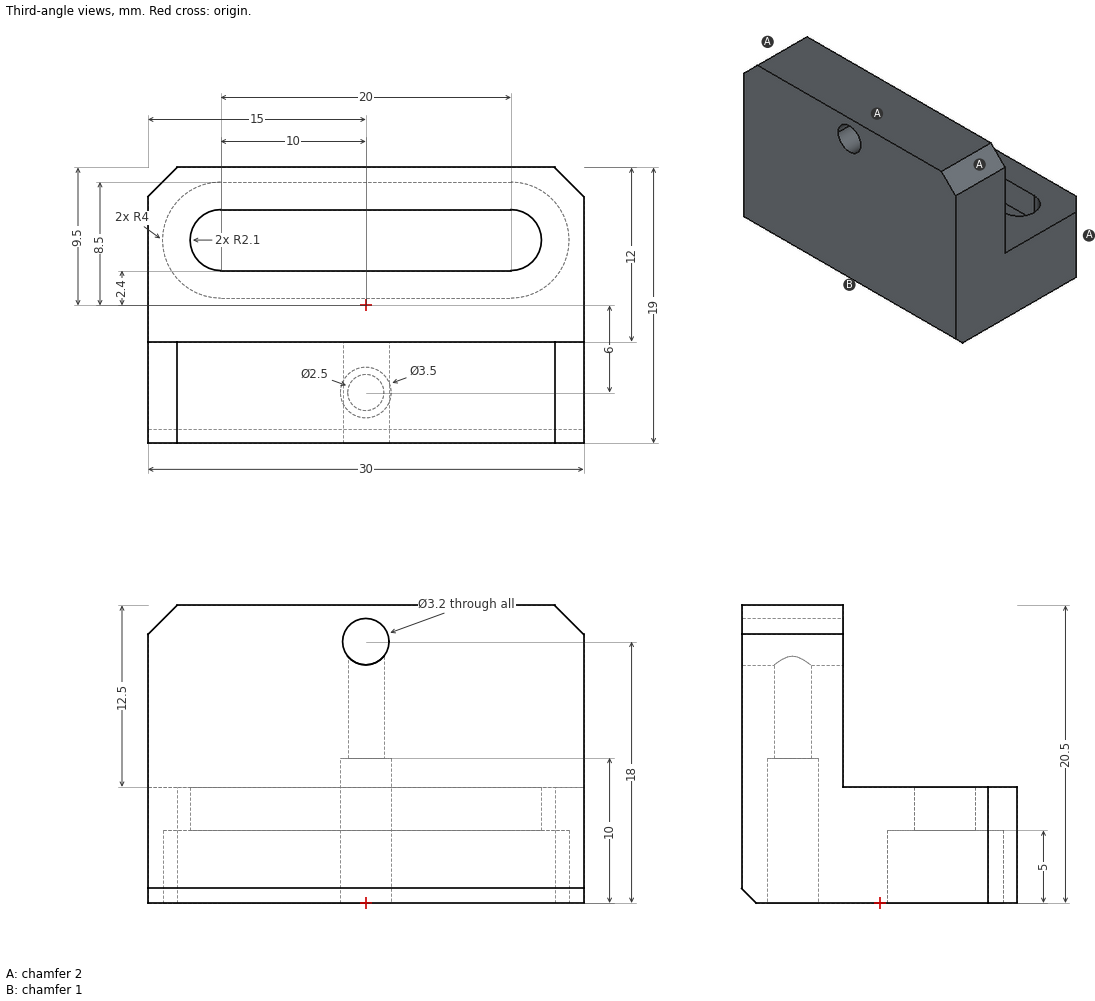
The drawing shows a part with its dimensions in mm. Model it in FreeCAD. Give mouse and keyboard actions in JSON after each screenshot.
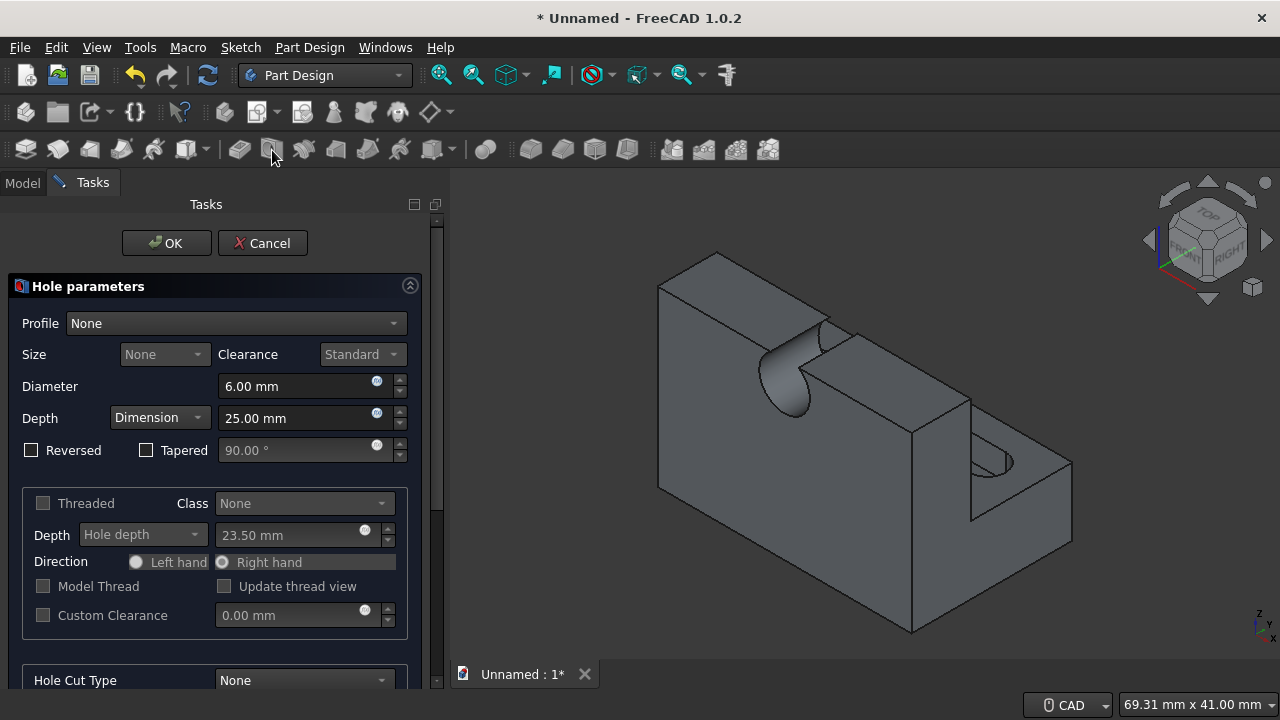
{"action": "triple_click", "coordinate": [305, 386]}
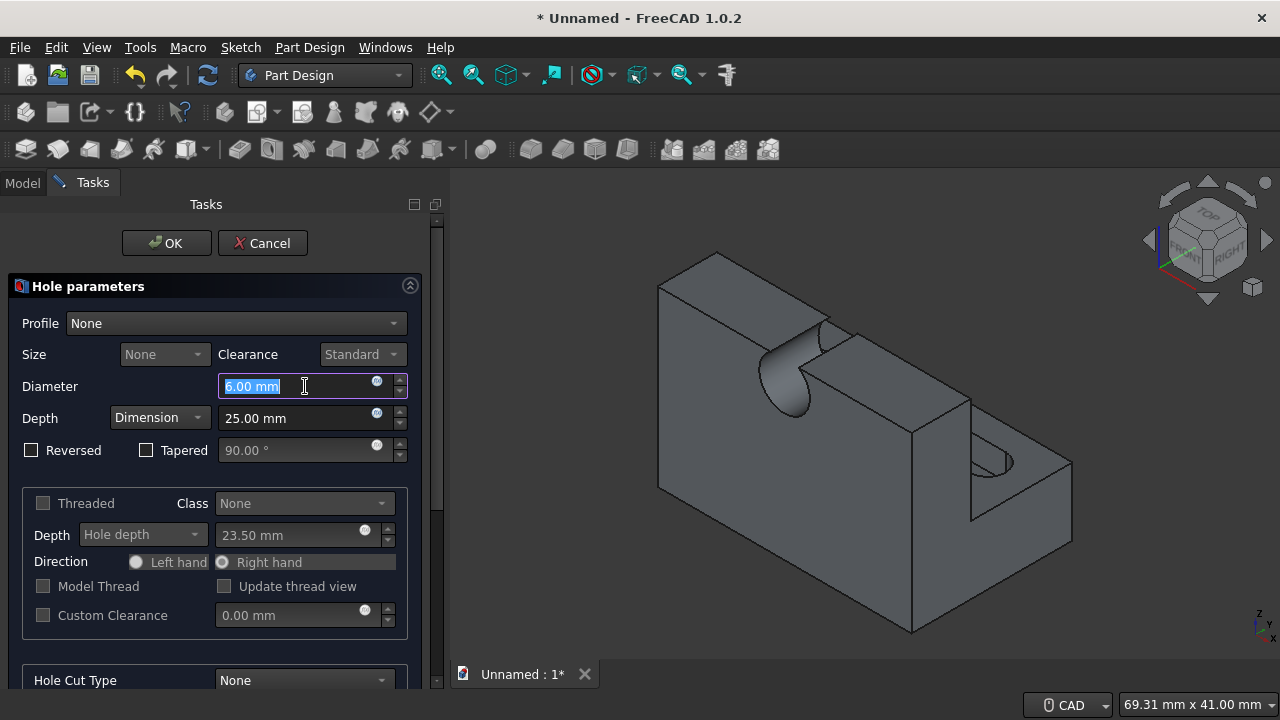
{"action": "type", "text": "3.2"}
{"action": "key", "text": "Tab"}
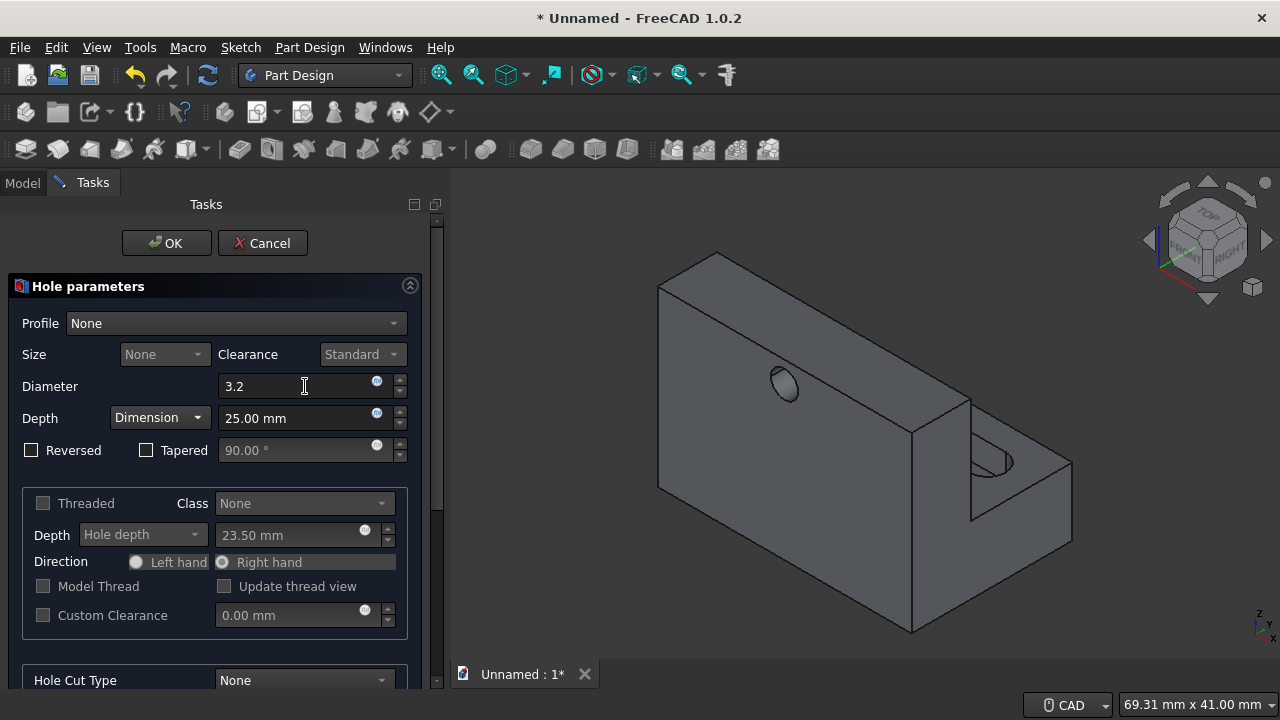
{"action": "left_click", "coordinate": [161, 418]}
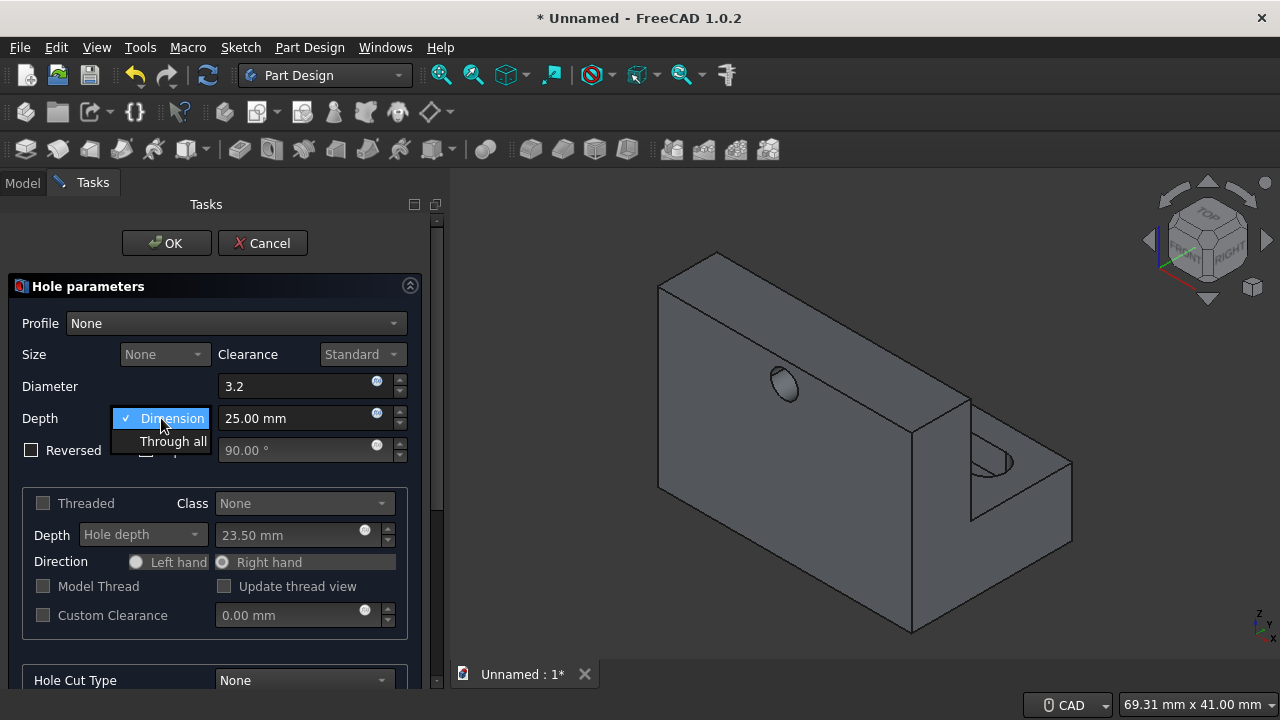
{"action": "left_click", "coordinate": [160, 442]}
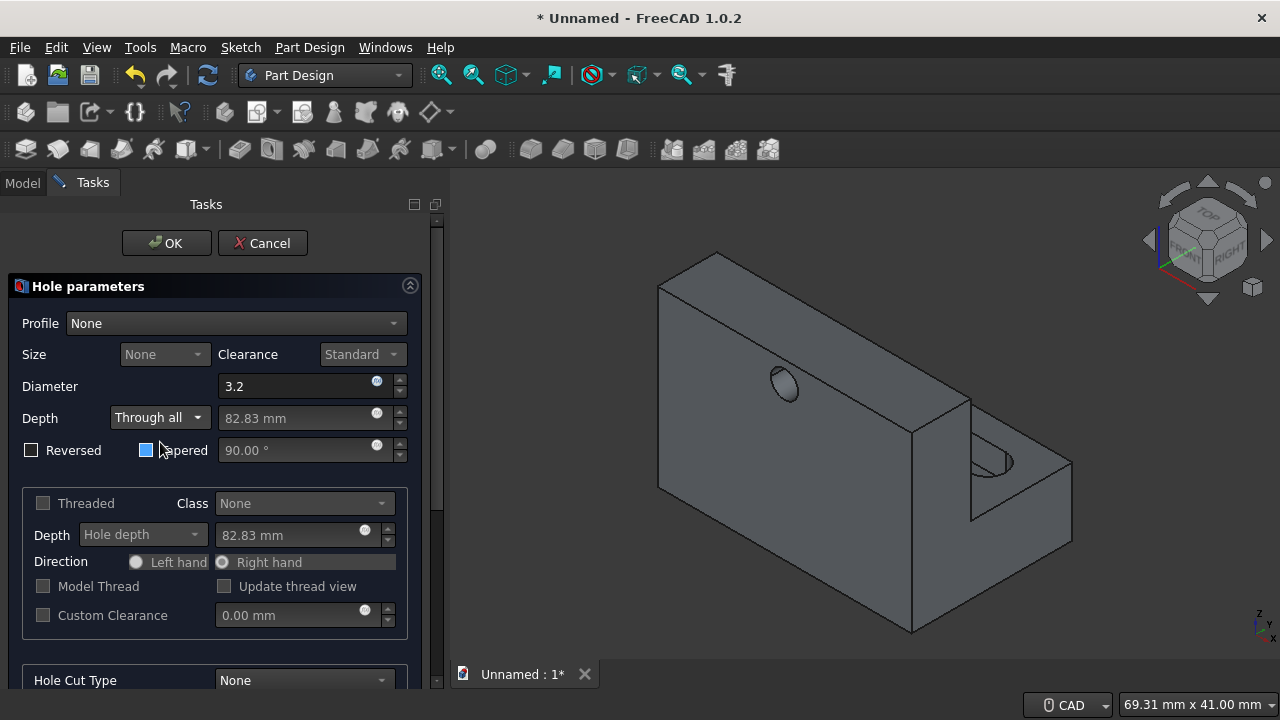
{"action": "left_click", "coordinate": [167, 243]}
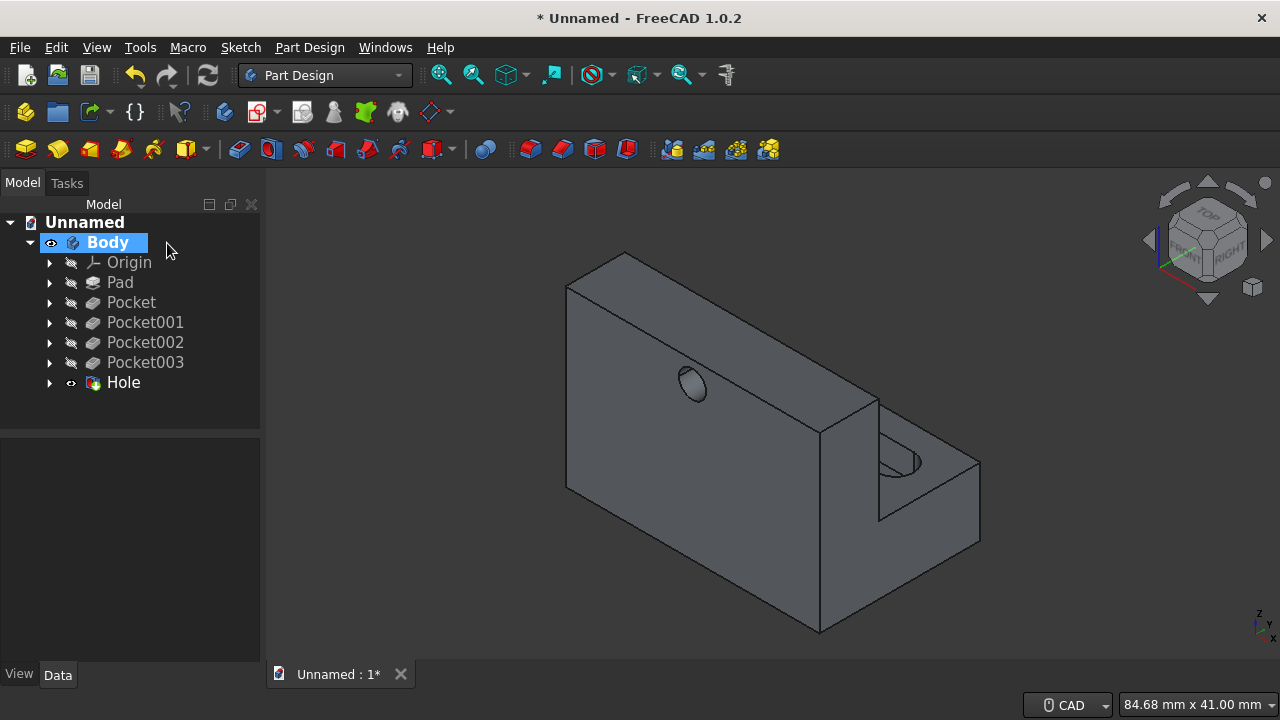
{"action": "key", "text": "5"}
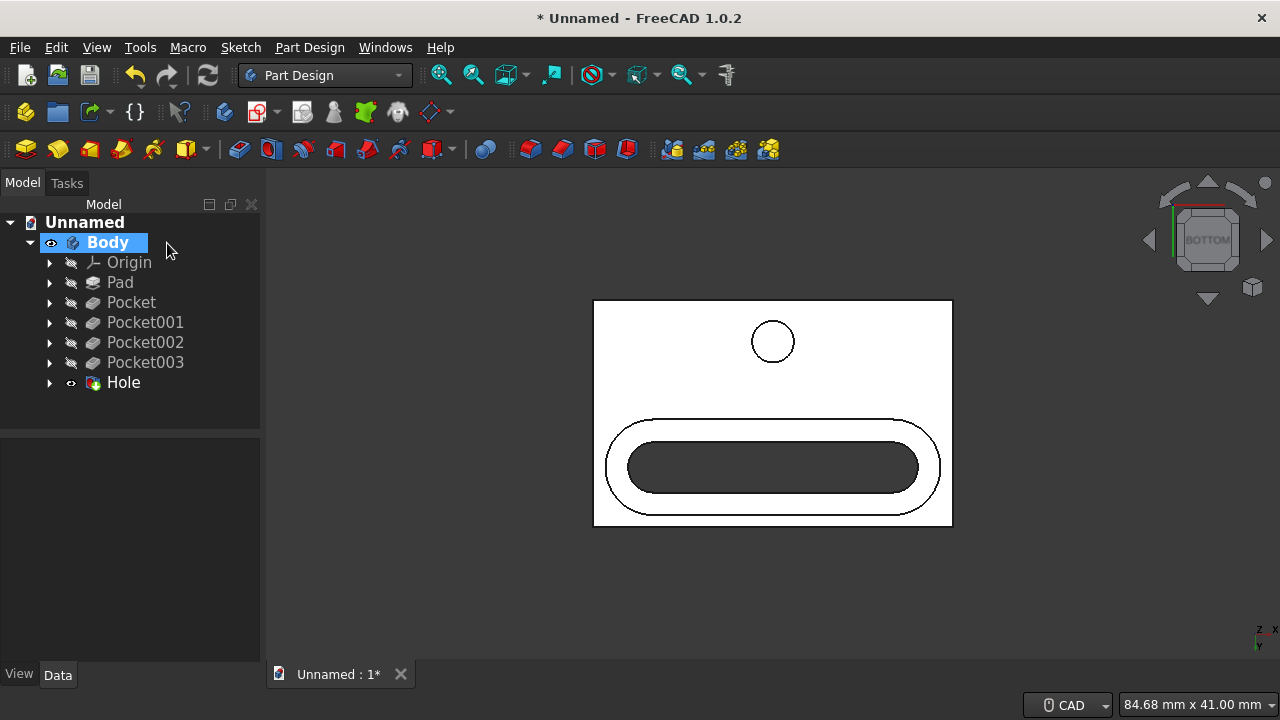
{"action": "left_click", "coordinate": [773, 341]}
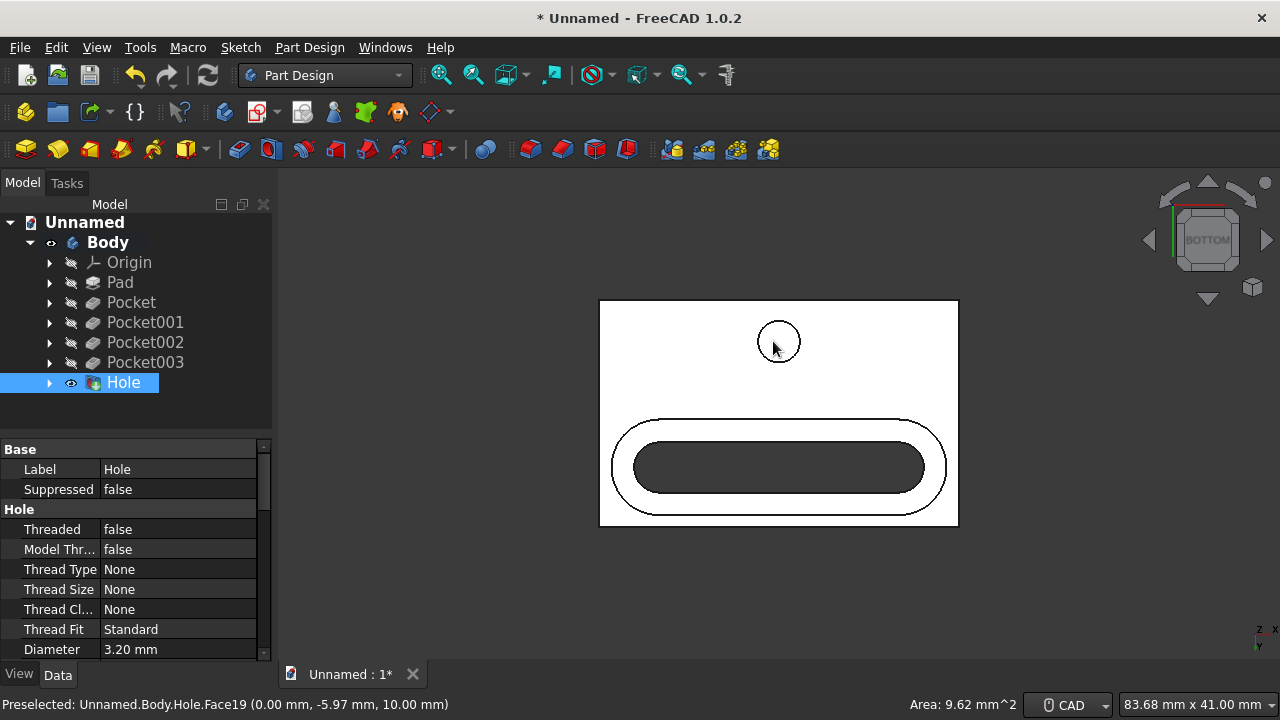
{"action": "left_click", "coordinate": [258, 112]}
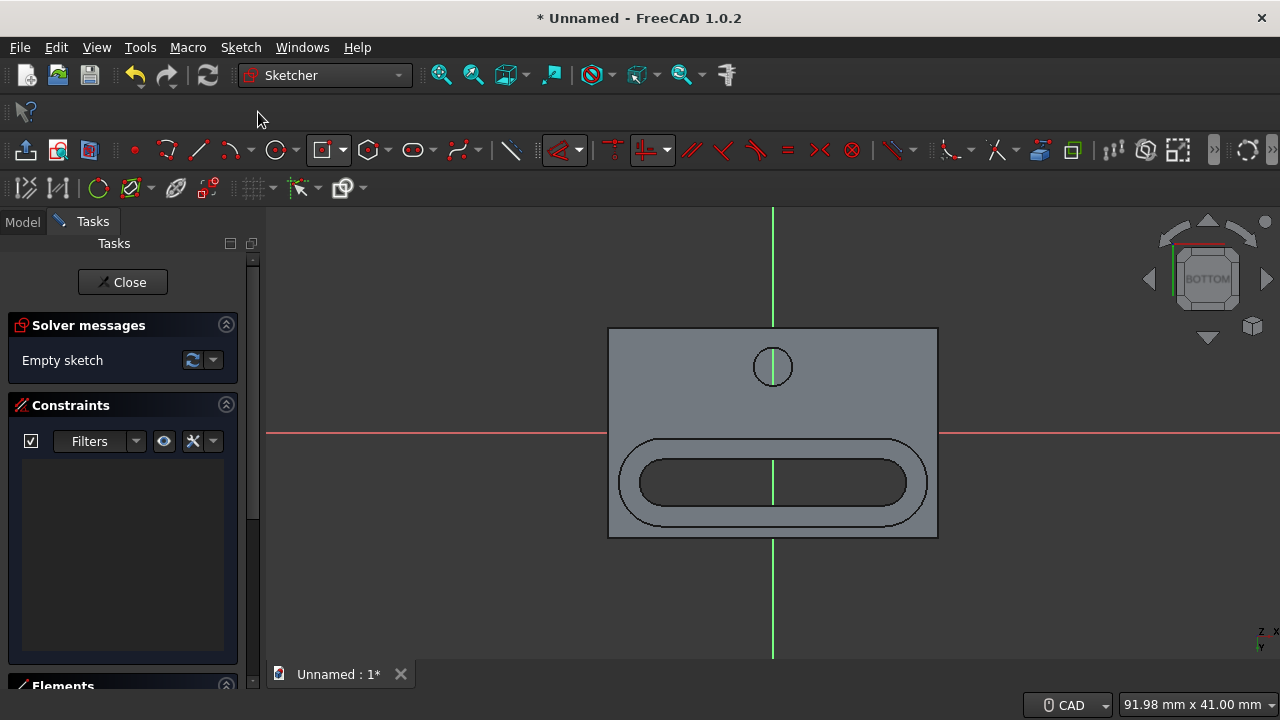
{"action": "left_click", "coordinate": [90, 150]}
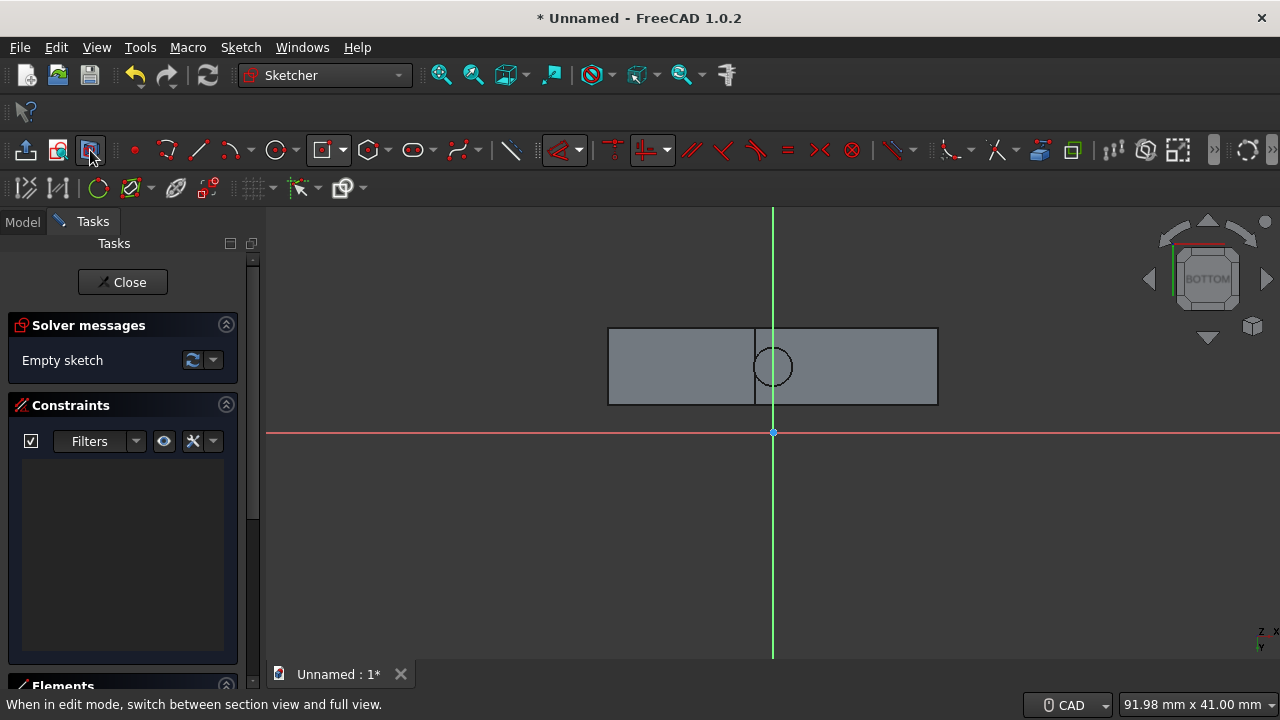
{"action": "scroll", "coordinate": [780, 360], "scroll_direction": "up", "scroll_amount": 12}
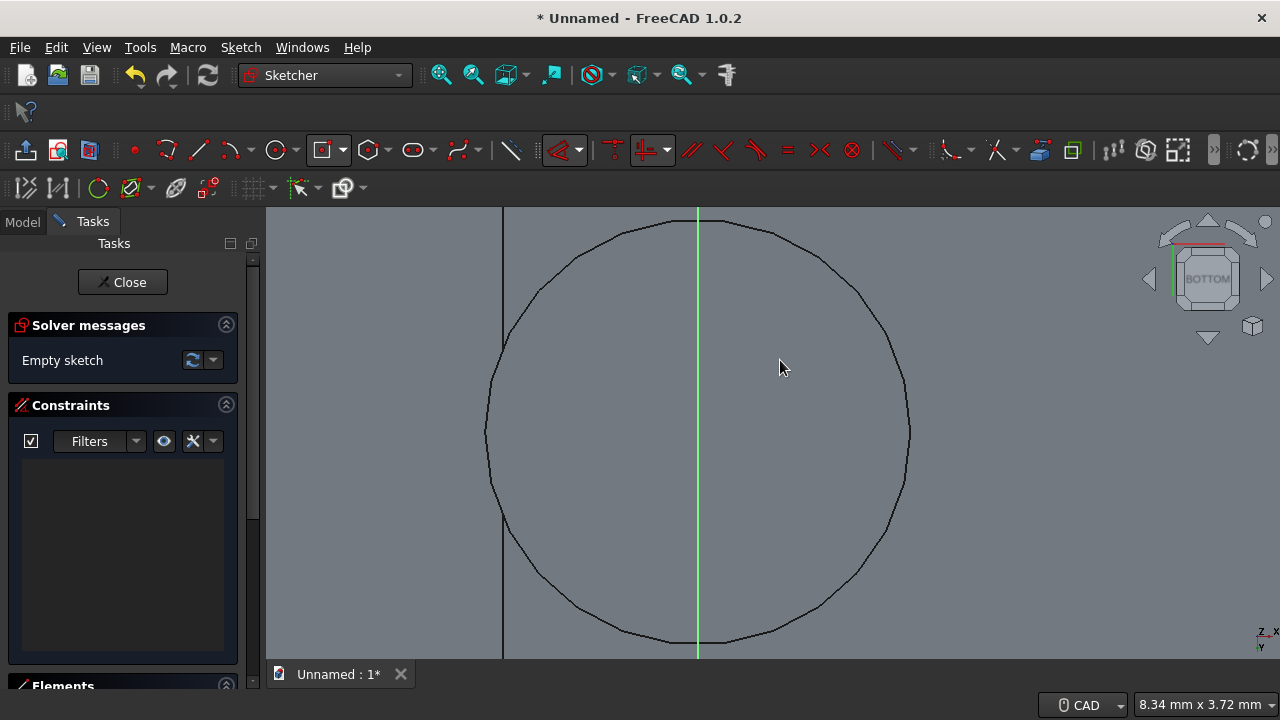
{"action": "key", "text": "g c"}